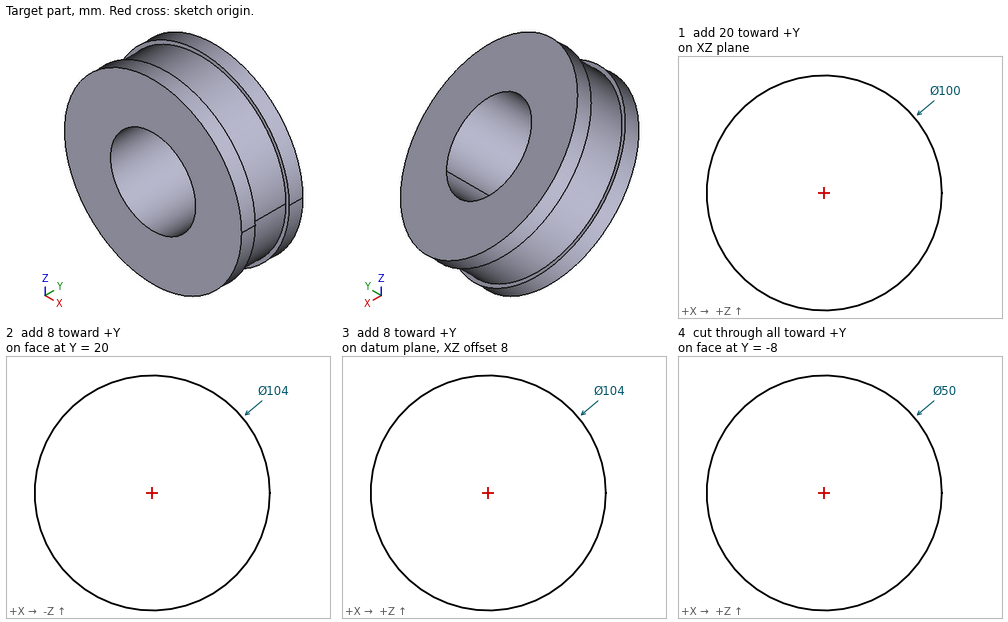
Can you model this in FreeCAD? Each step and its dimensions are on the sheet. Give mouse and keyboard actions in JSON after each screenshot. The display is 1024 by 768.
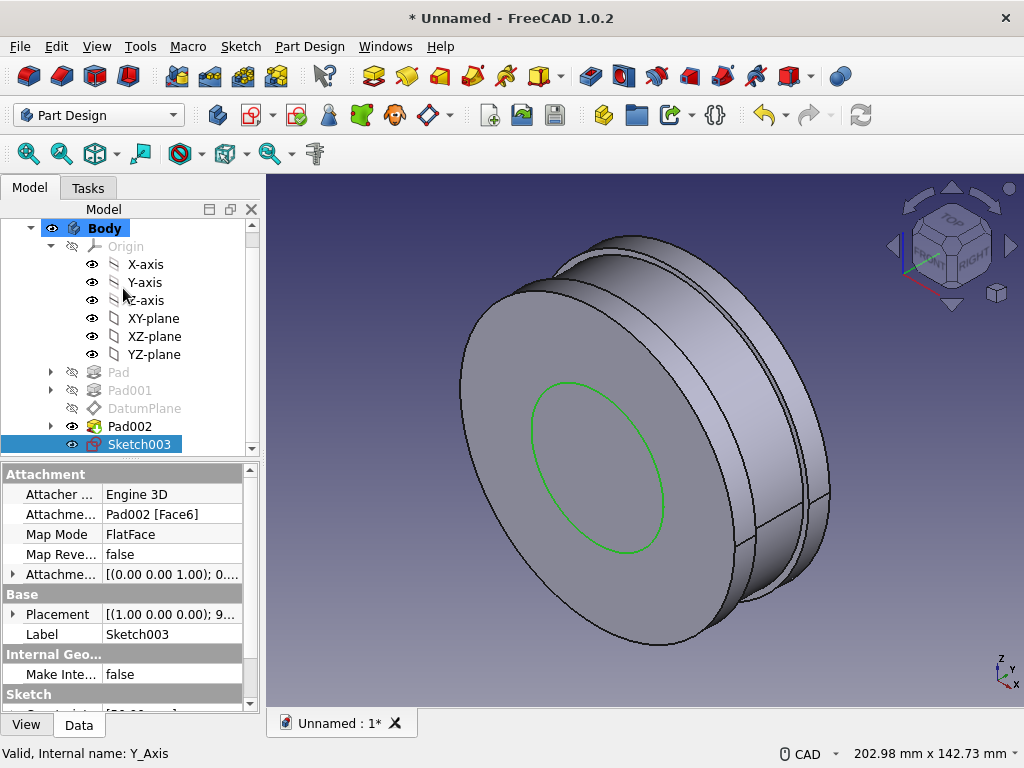
{"action": "left_click", "coordinate": [591, 76]}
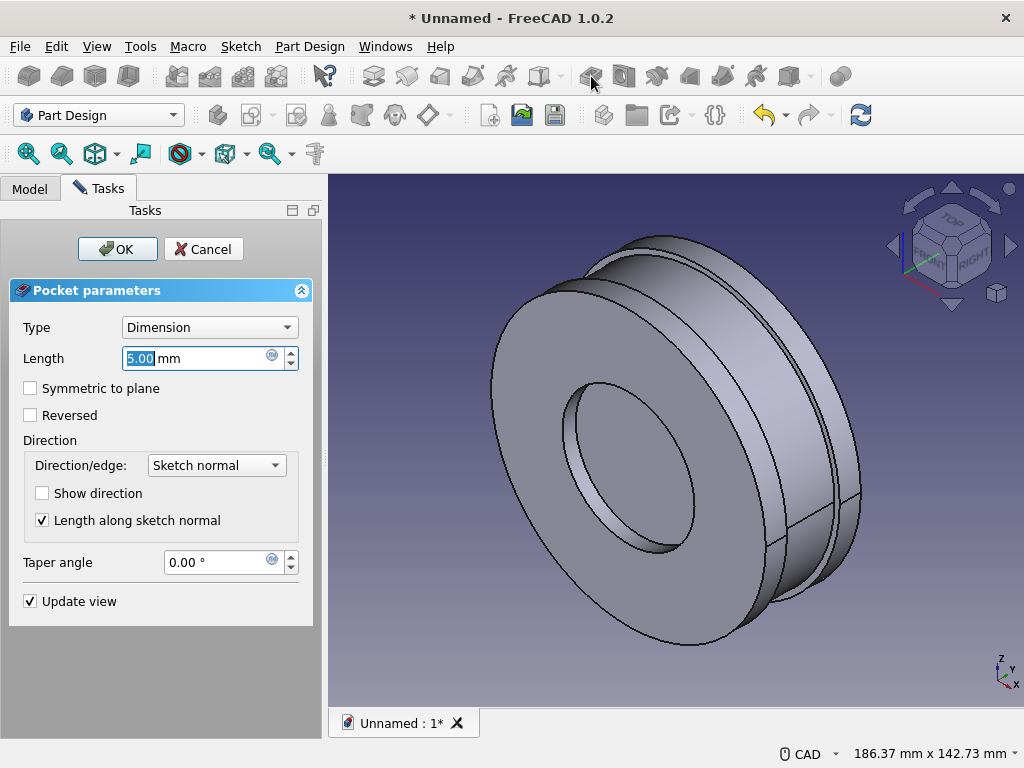
{"action": "left_click", "coordinate": [210, 328]}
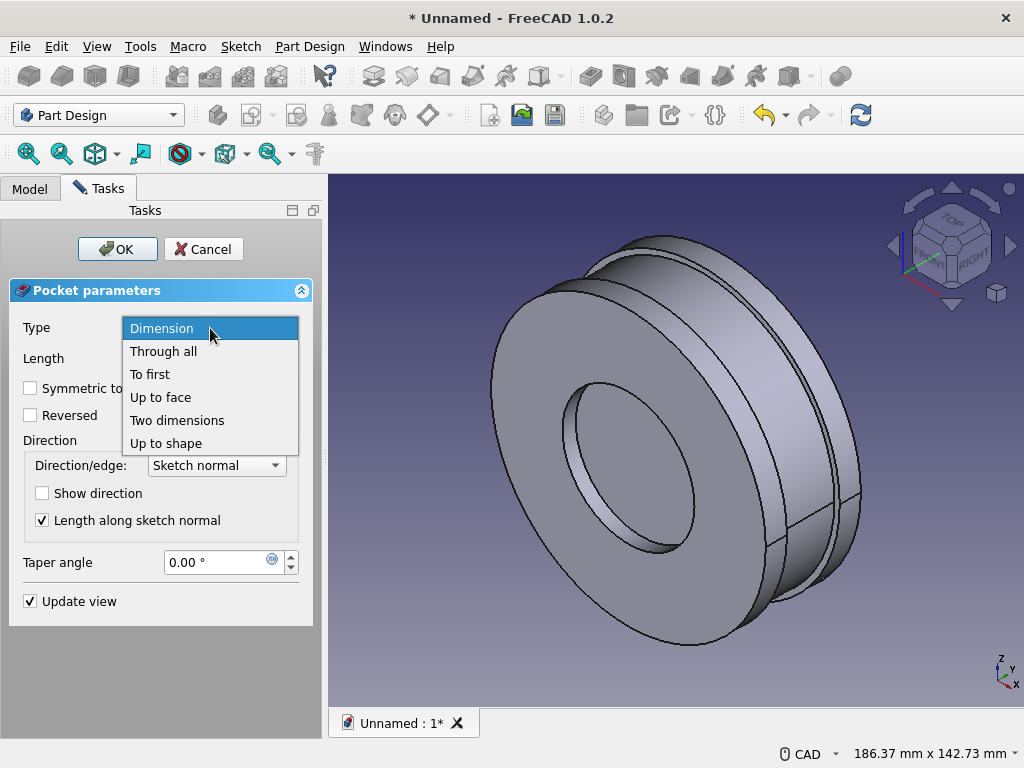
{"action": "left_click", "coordinate": [208, 352]}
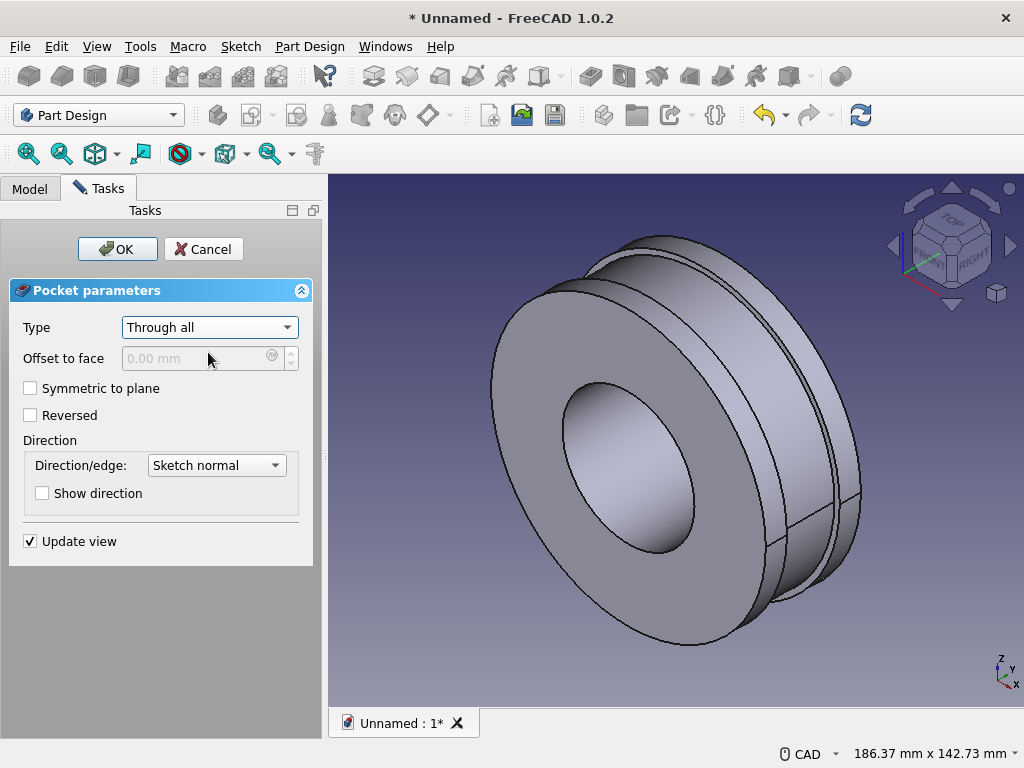
{"action": "left_click", "coordinate": [118, 249]}